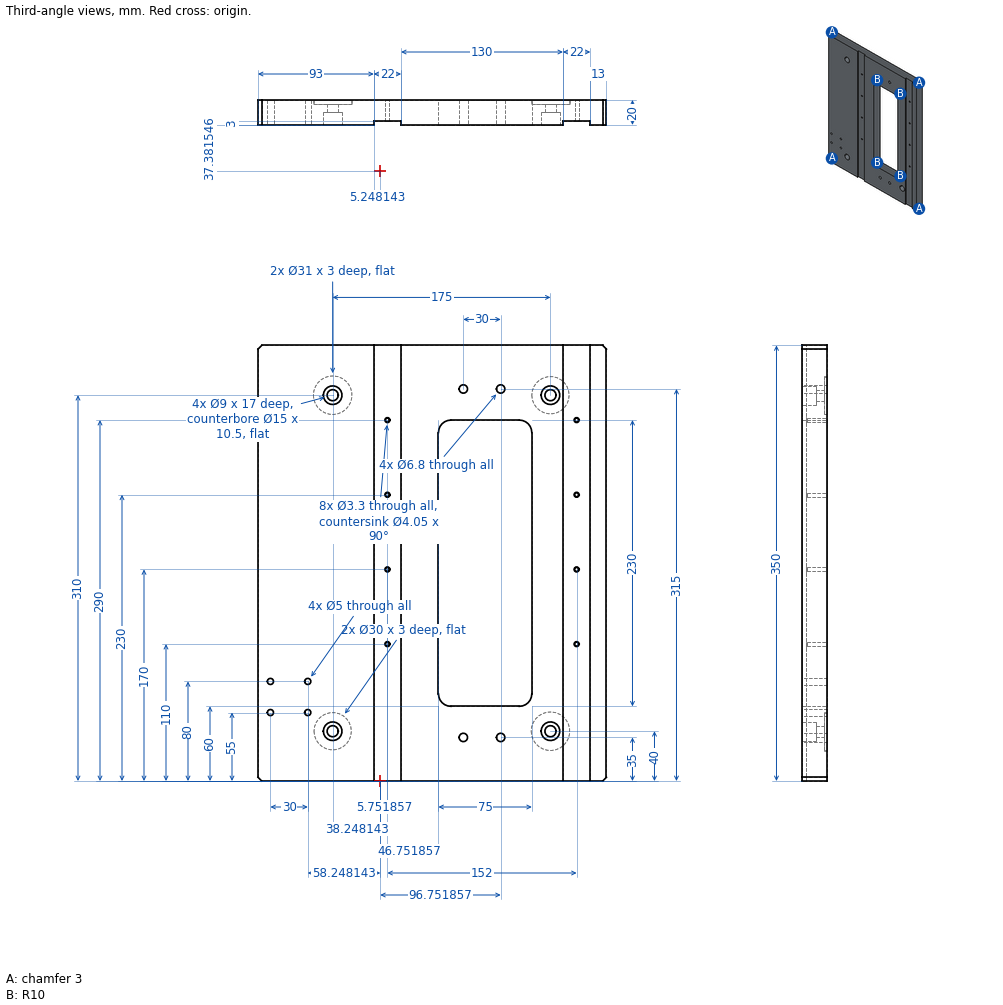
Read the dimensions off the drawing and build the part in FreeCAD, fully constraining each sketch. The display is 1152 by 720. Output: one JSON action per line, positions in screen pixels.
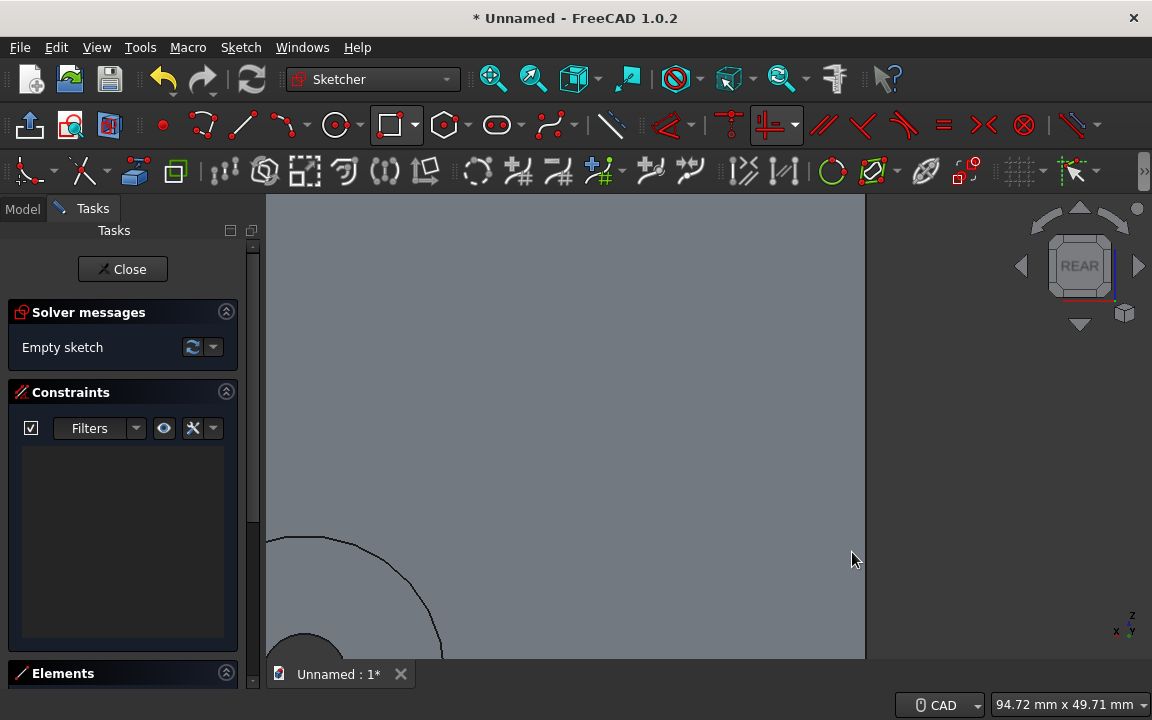
{"action": "left_click", "coordinate": [336, 126]}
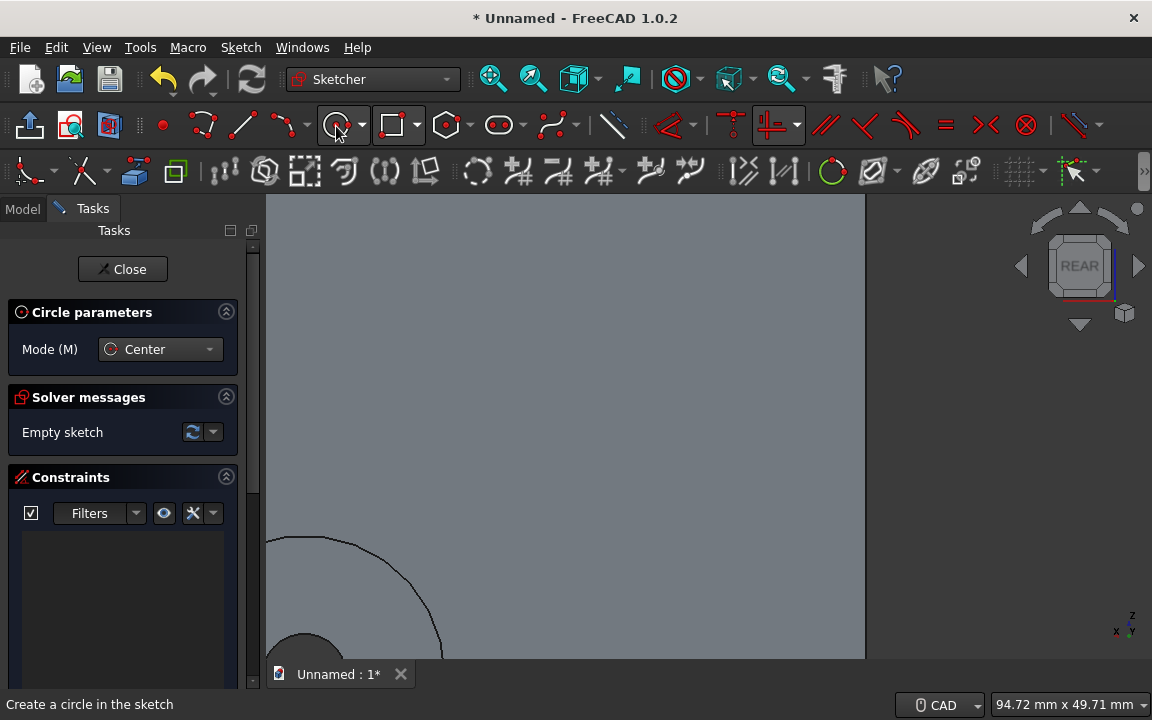
{"action": "left_click", "coordinate": [491, 302]}
{"action": "mouse_move", "coordinate": [508, 285]}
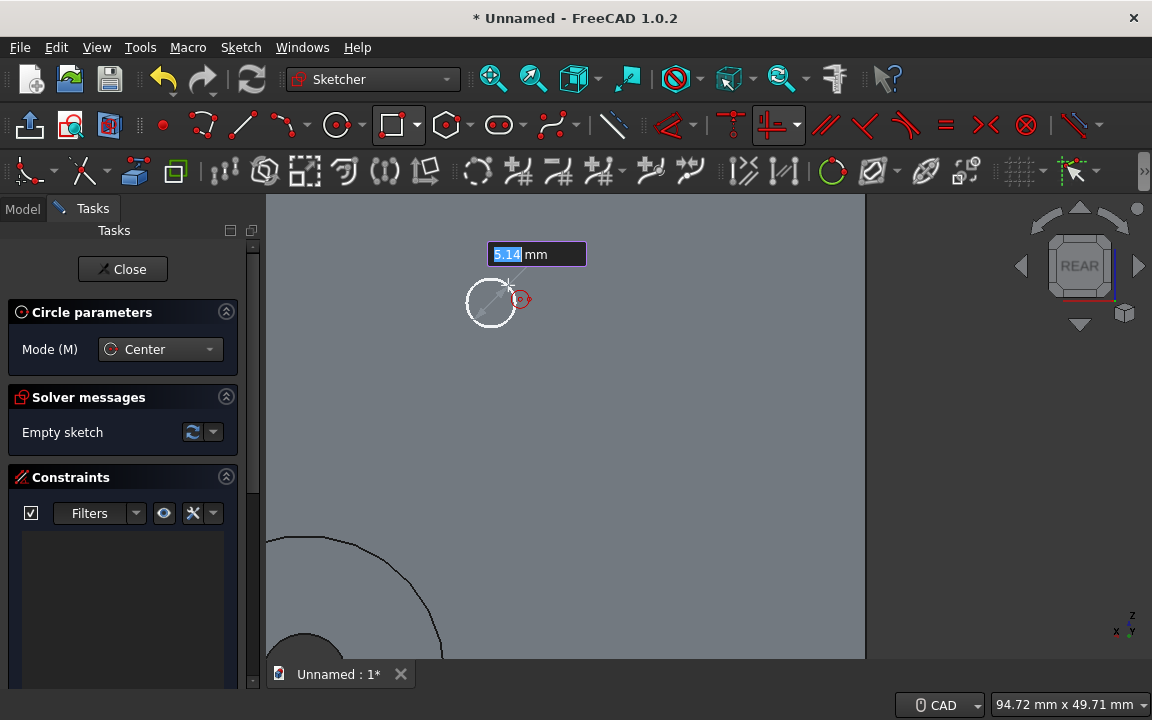
{"action": "type", "text": "5"}
{"action": "key", "text": "Return"}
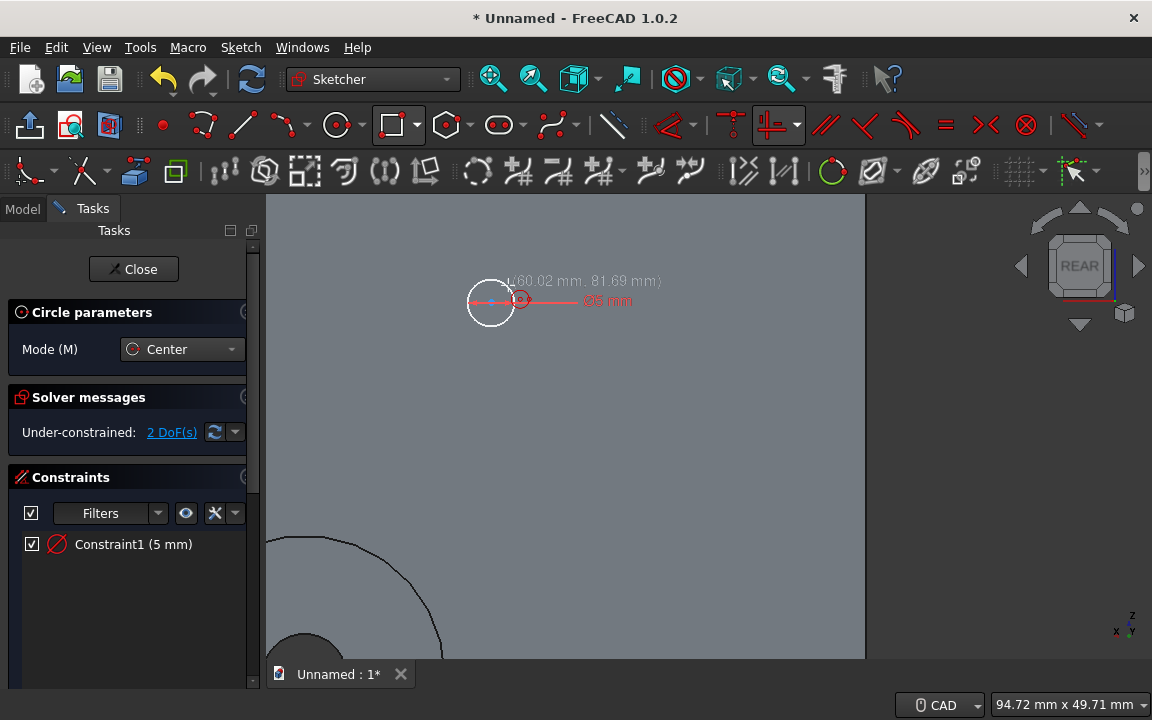
{"action": "left_click", "coordinate": [491, 536]}
{"action": "mouse_move", "coordinate": [508, 519]}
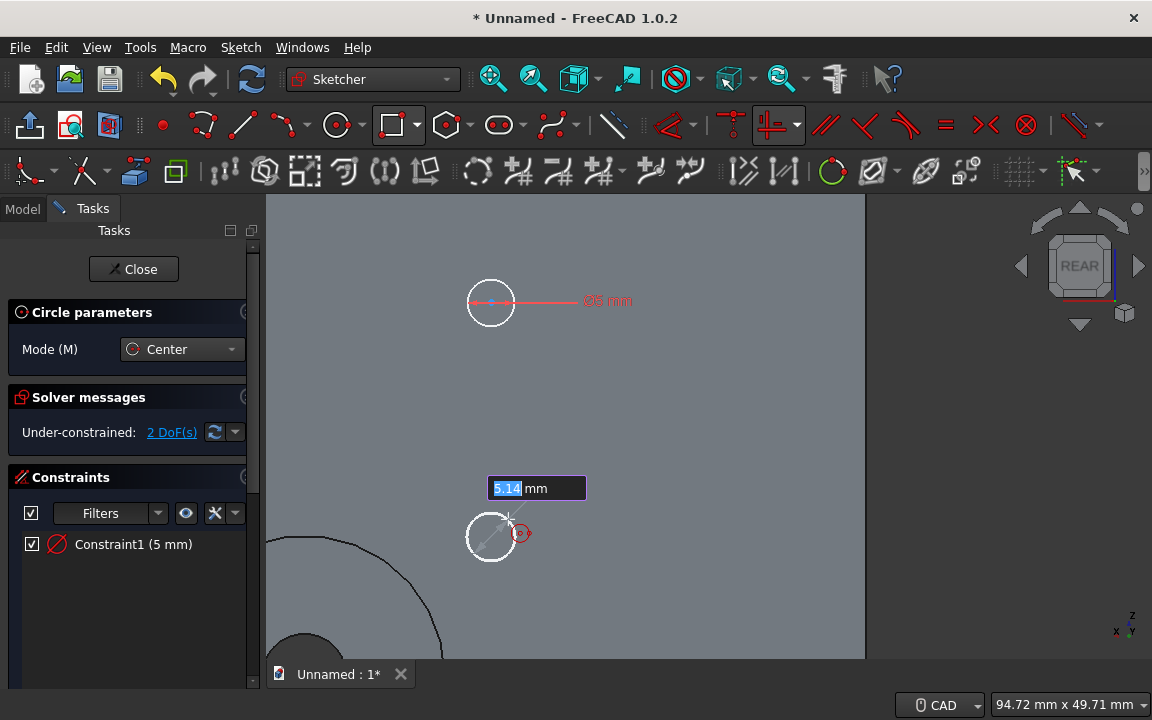
{"action": "type", "text": "5"}
{"action": "key", "text": "Return"}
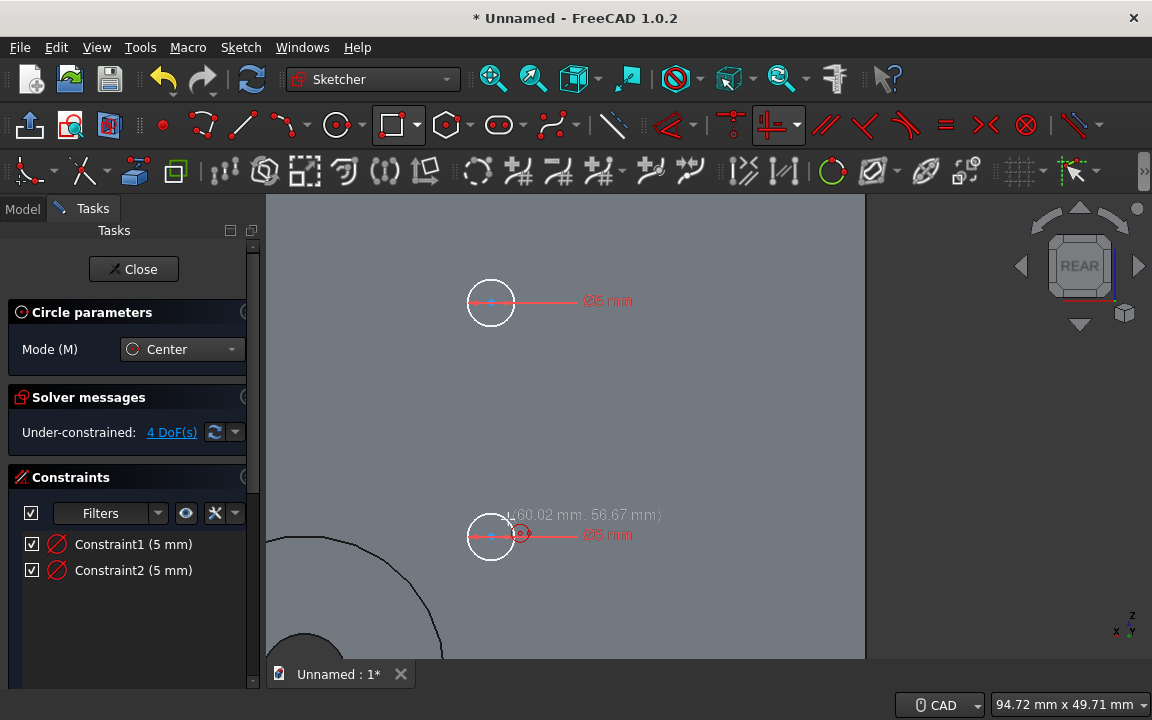
{"action": "left_click", "coordinate": [772, 536]}
{"action": "mouse_move", "coordinate": [789, 519]}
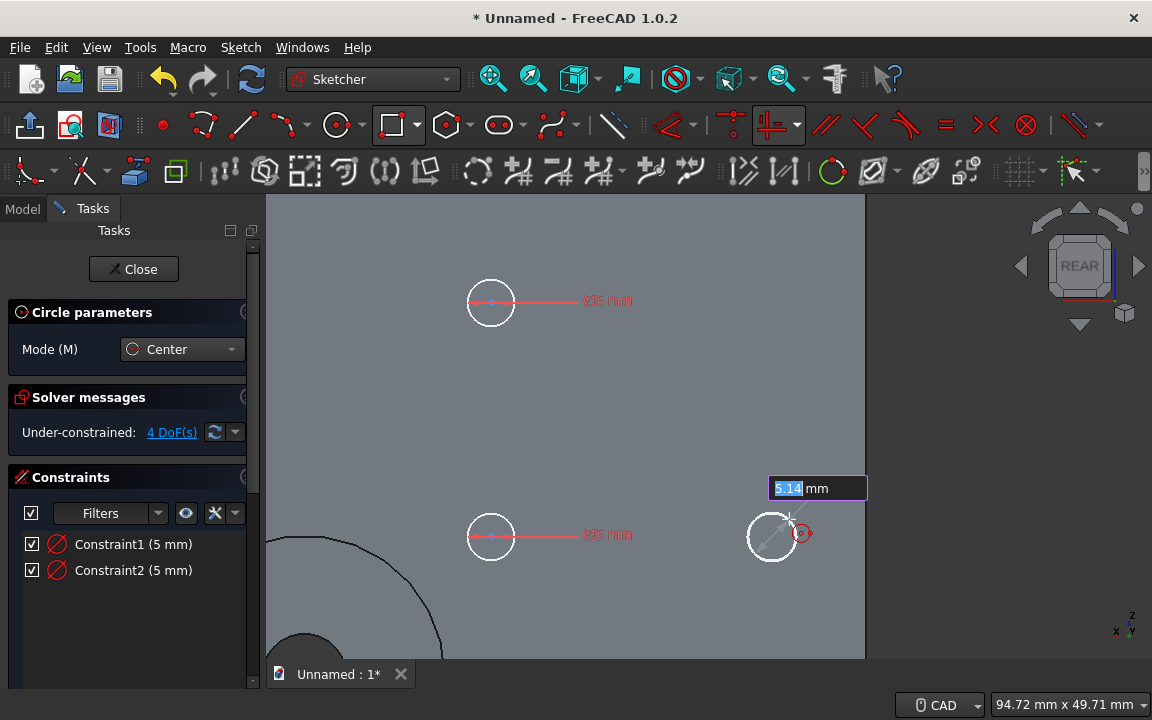
{"action": "type", "text": "5"}
{"action": "key", "text": "Return"}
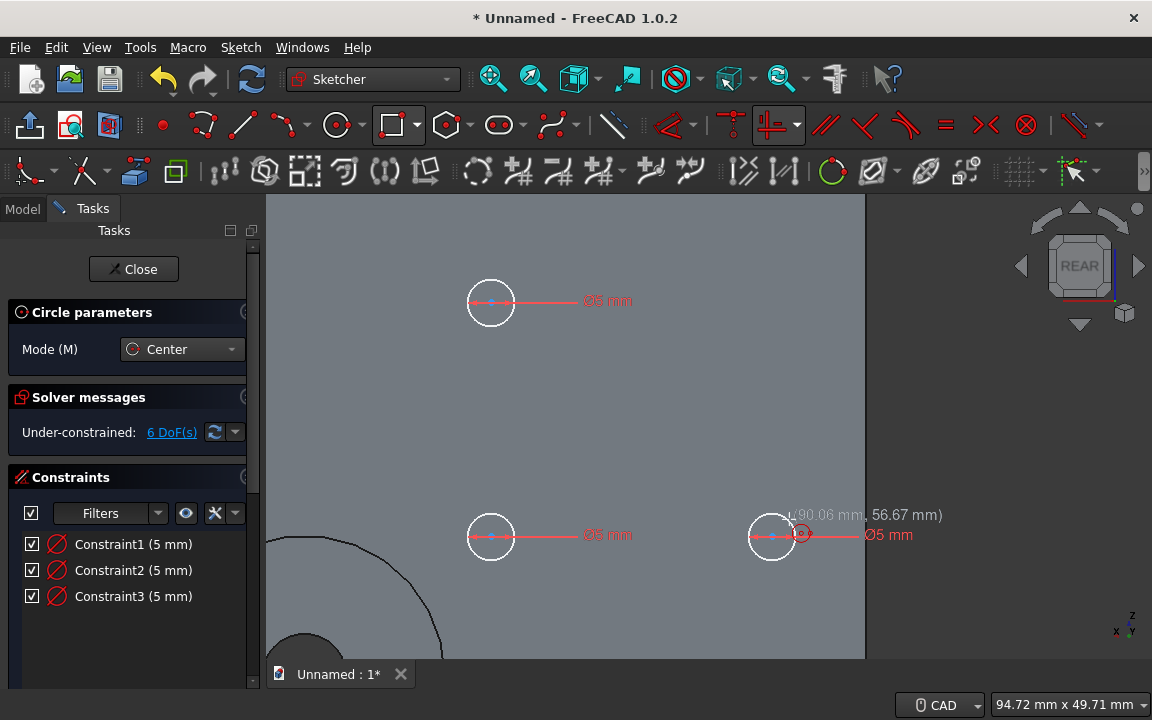
{"action": "left_click", "coordinate": [772, 302]}
{"action": "mouse_move", "coordinate": [789, 285]}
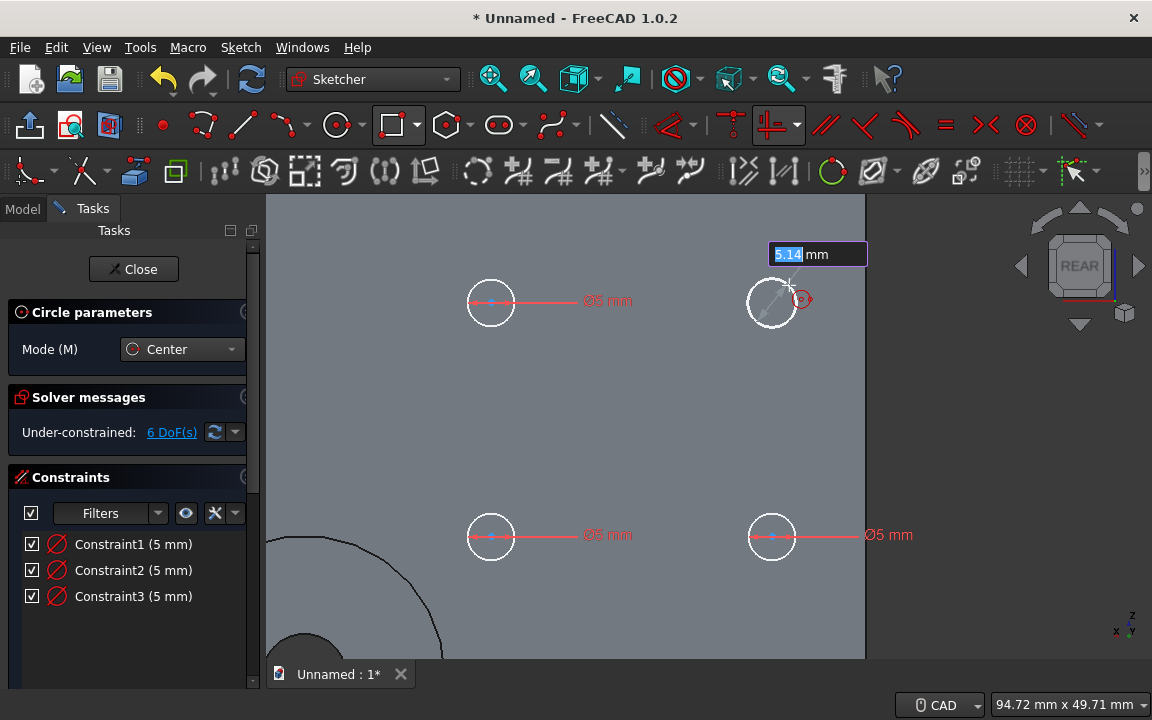
{"action": "type", "text": "5"}
{"action": "key", "text": "Return"}
{"action": "key", "text": "Escape"}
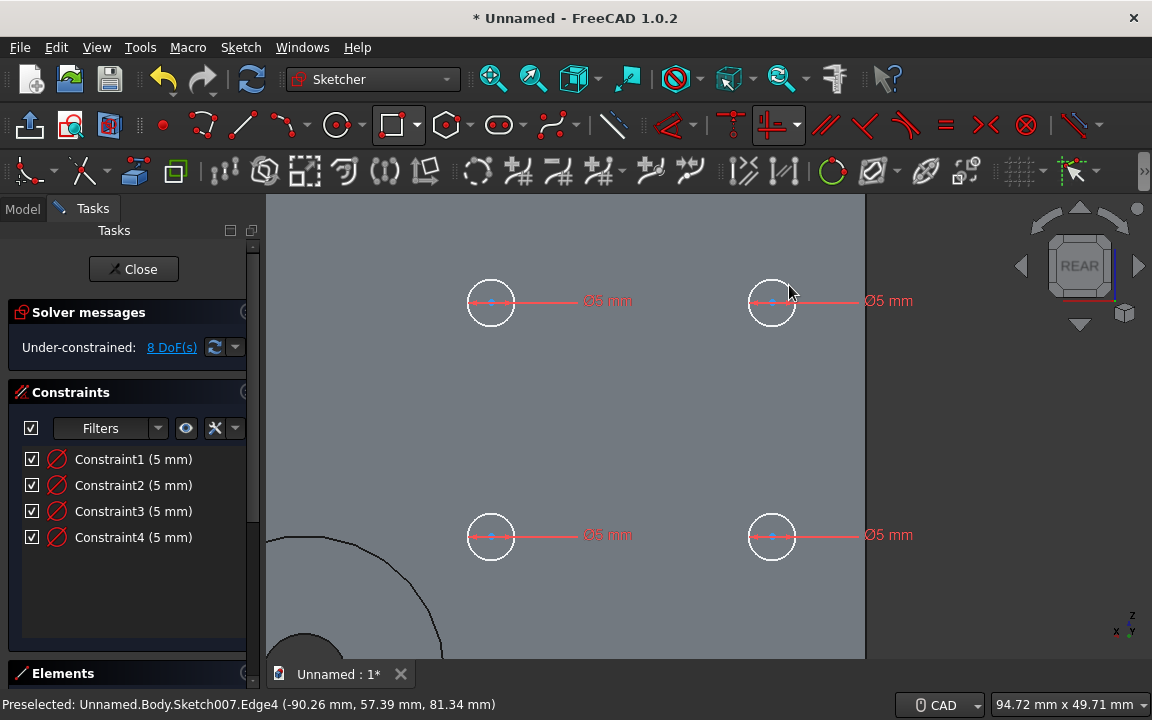
{"action": "left_click", "coordinate": [491, 303]}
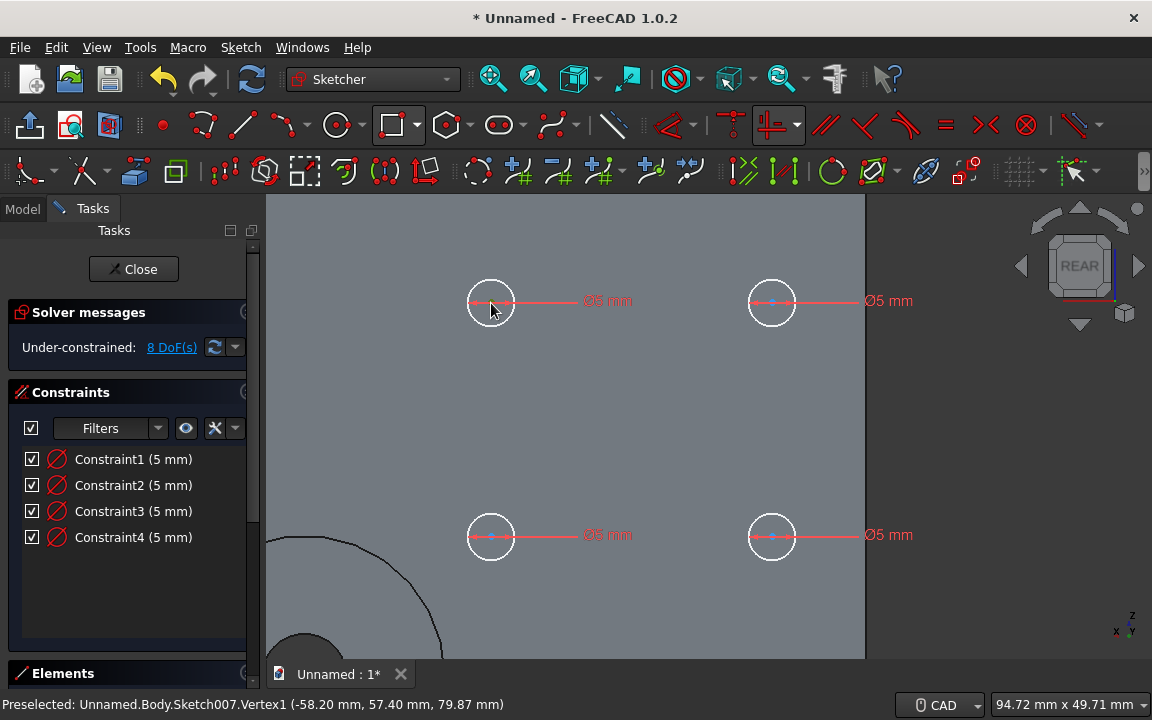
{"action": "left_click", "coordinate": [491, 537]}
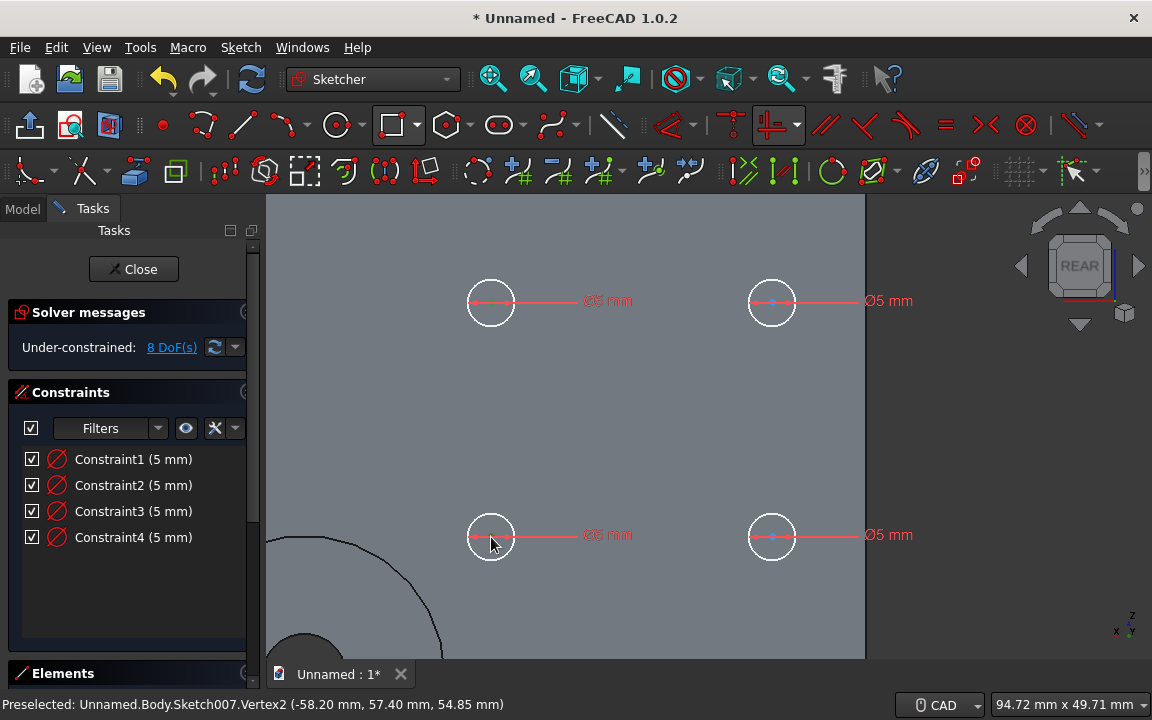
{"action": "left_click", "coordinate": [800, 126]}